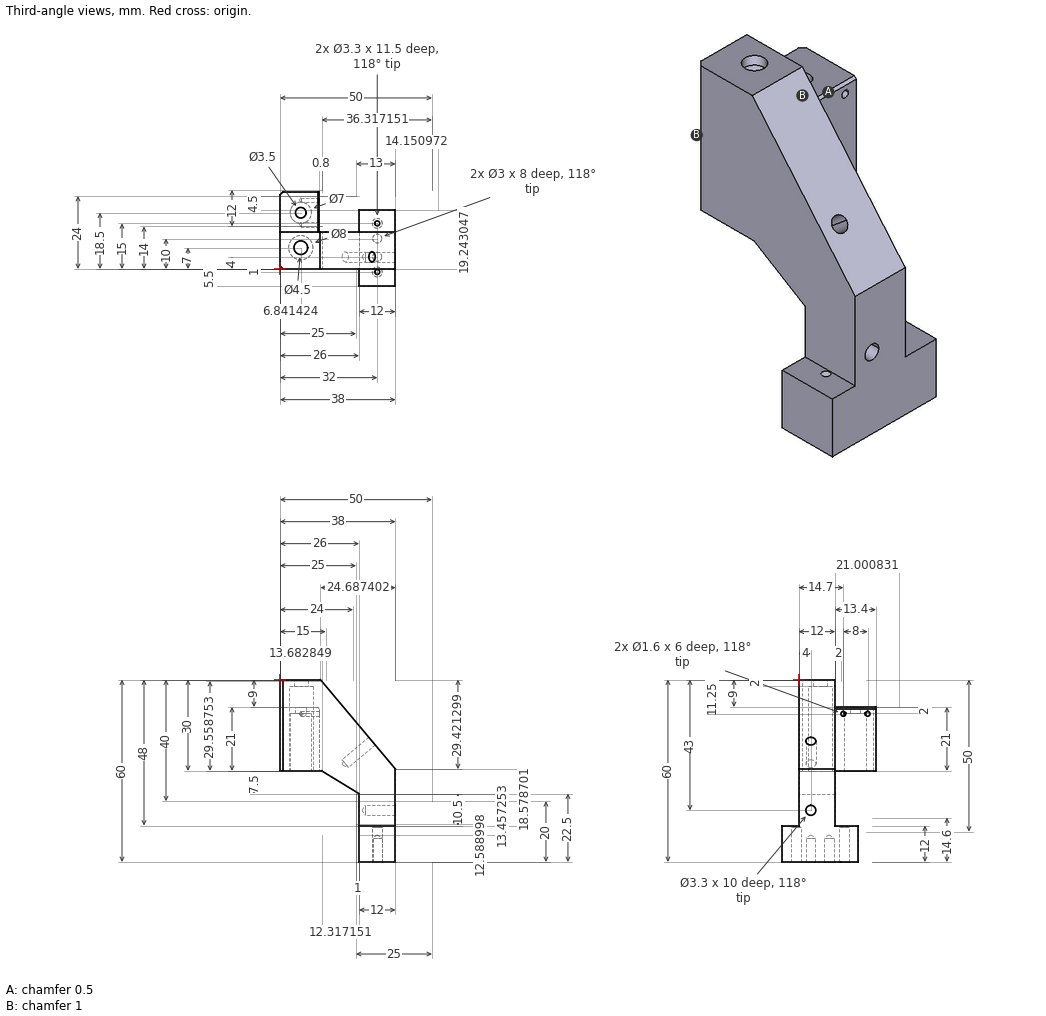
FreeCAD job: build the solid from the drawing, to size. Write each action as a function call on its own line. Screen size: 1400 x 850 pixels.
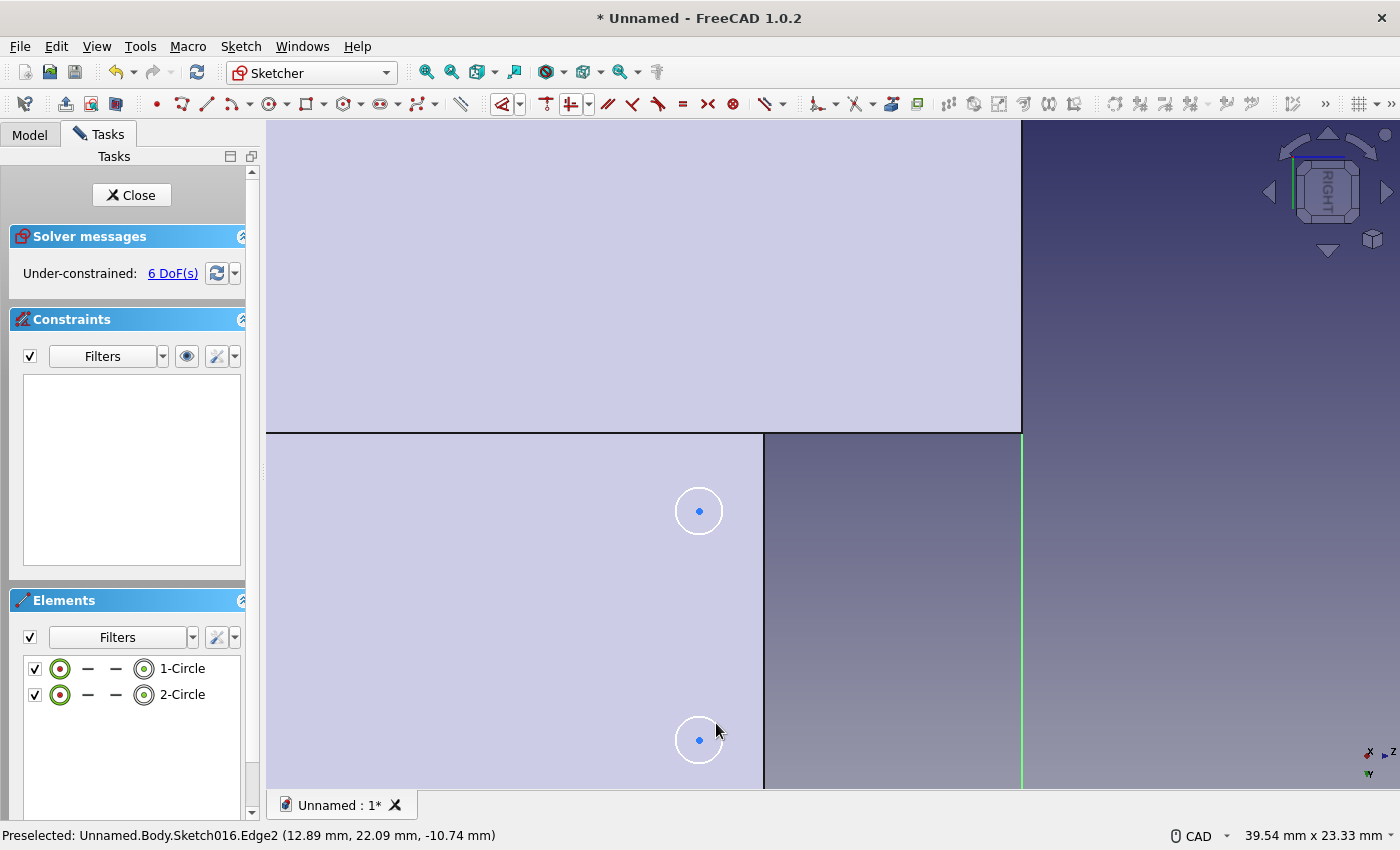
click(715, 494)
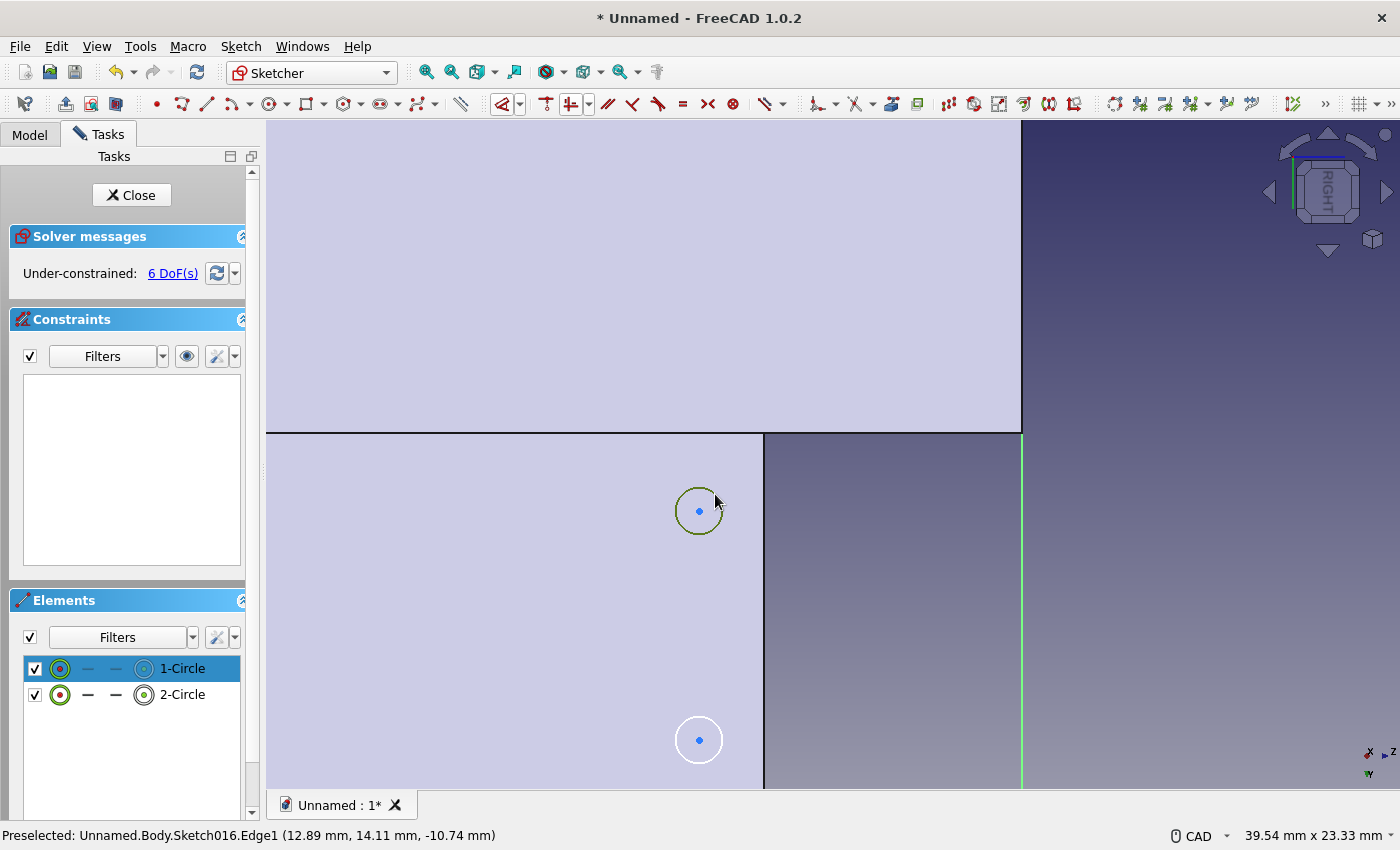
click(715, 723)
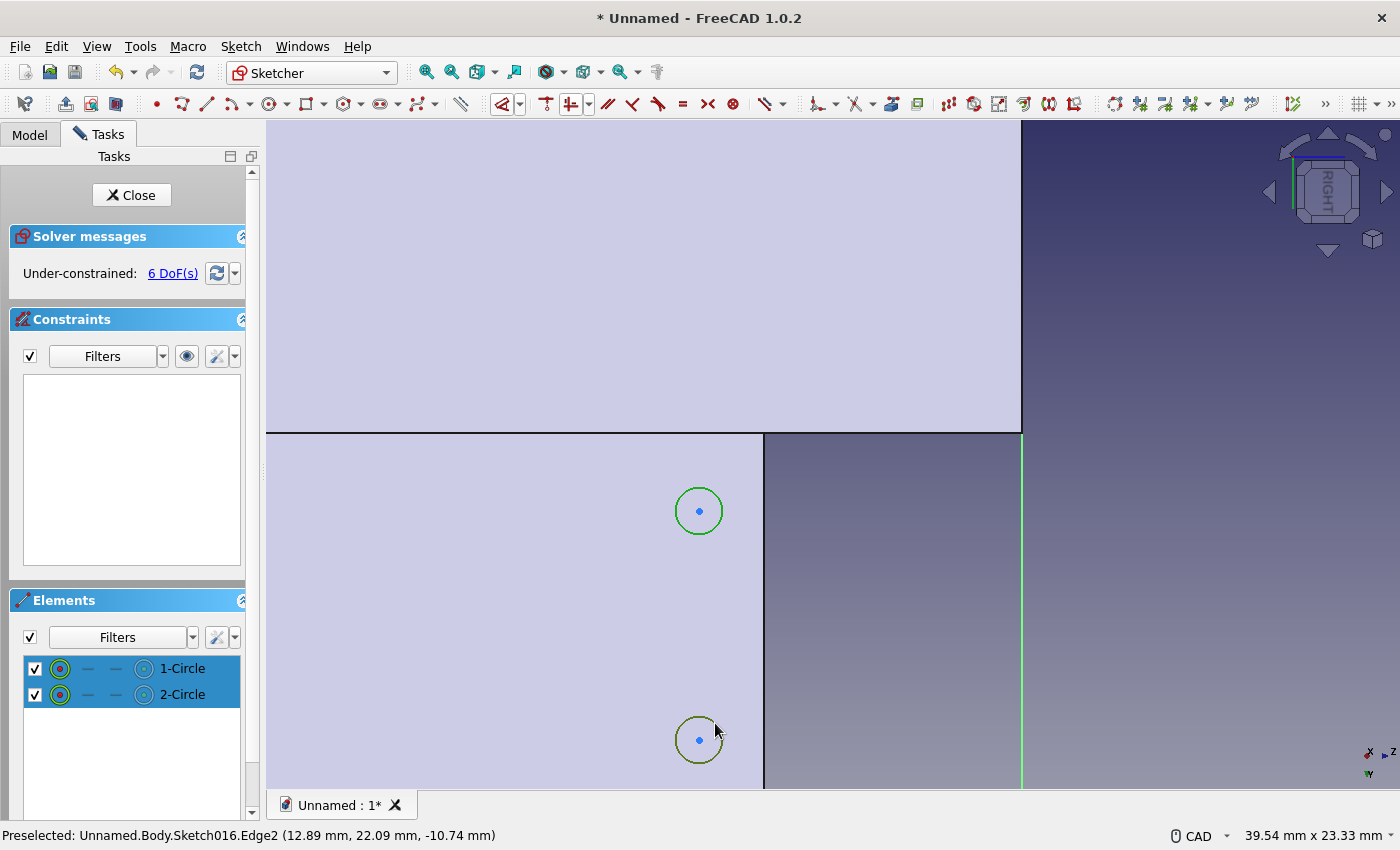
click(683, 104)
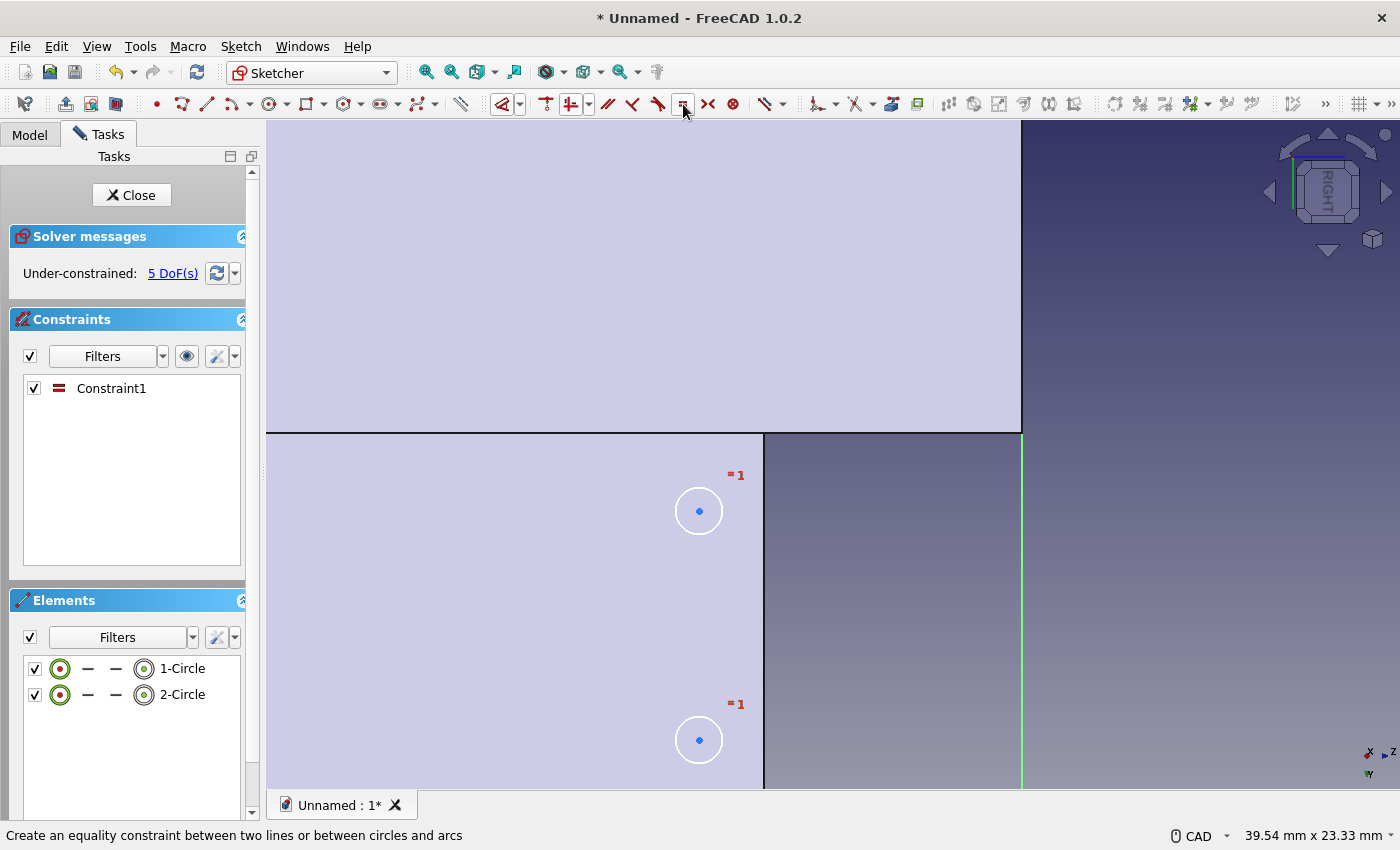
click(699, 511)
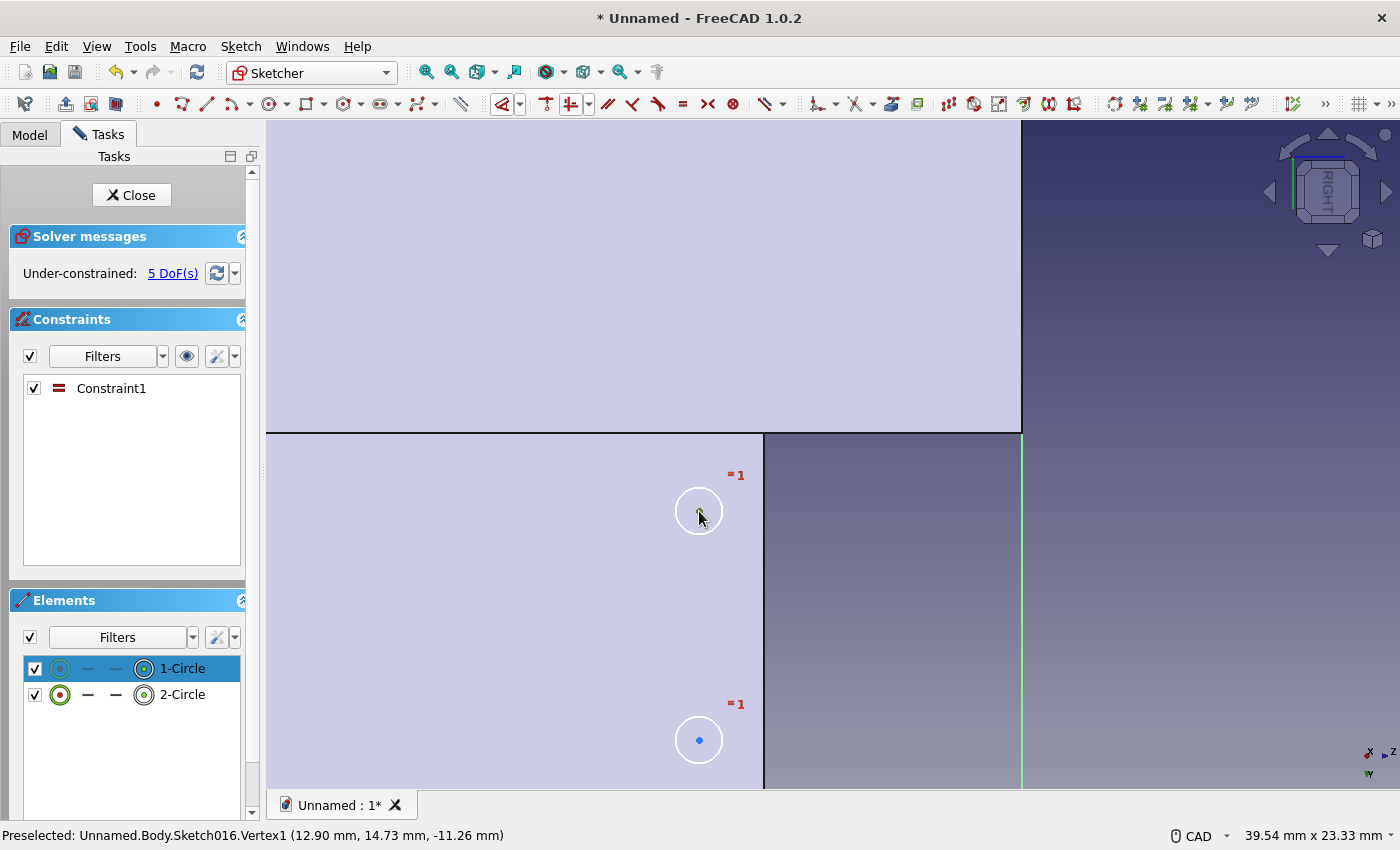
click(699, 740)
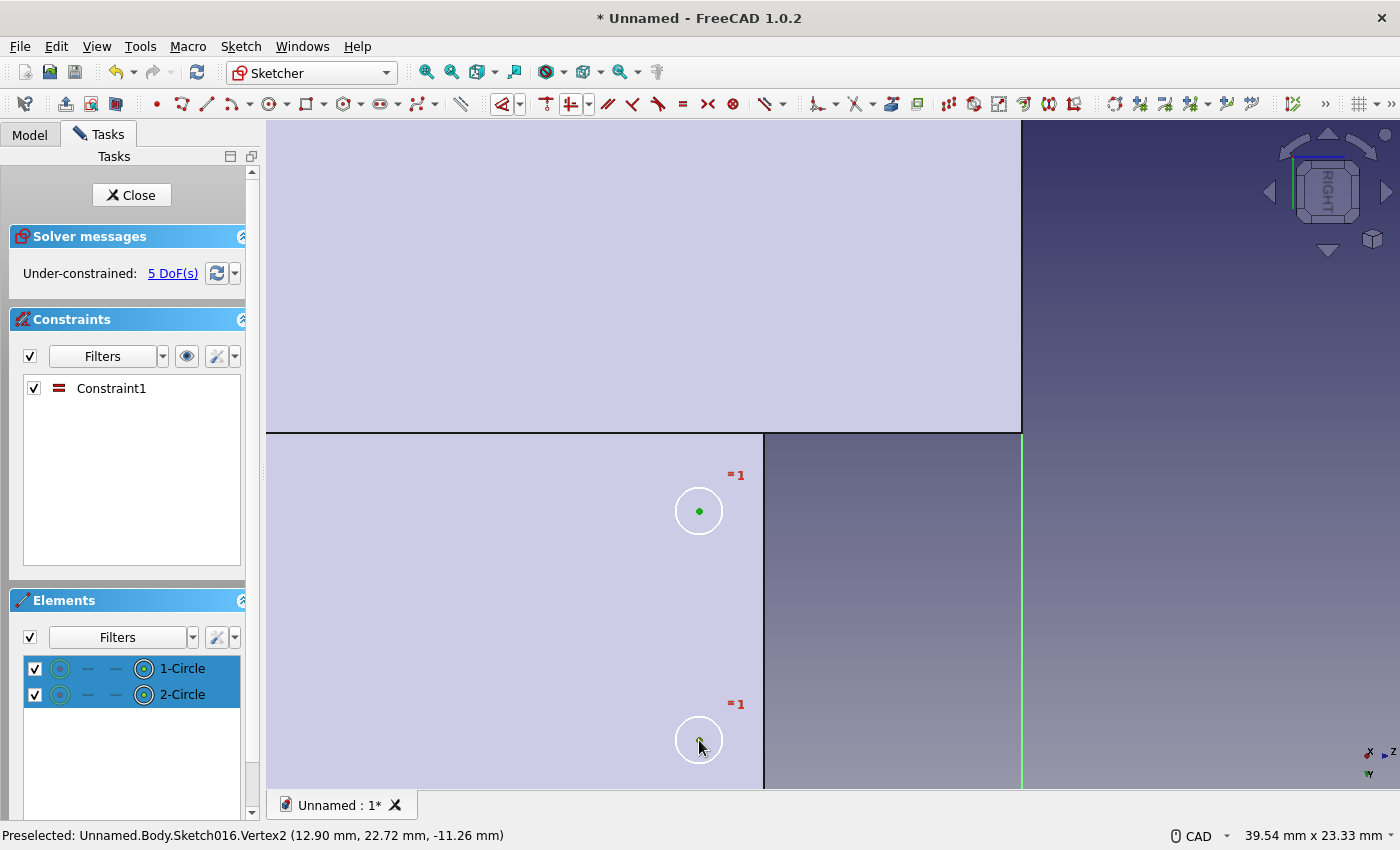
key(v)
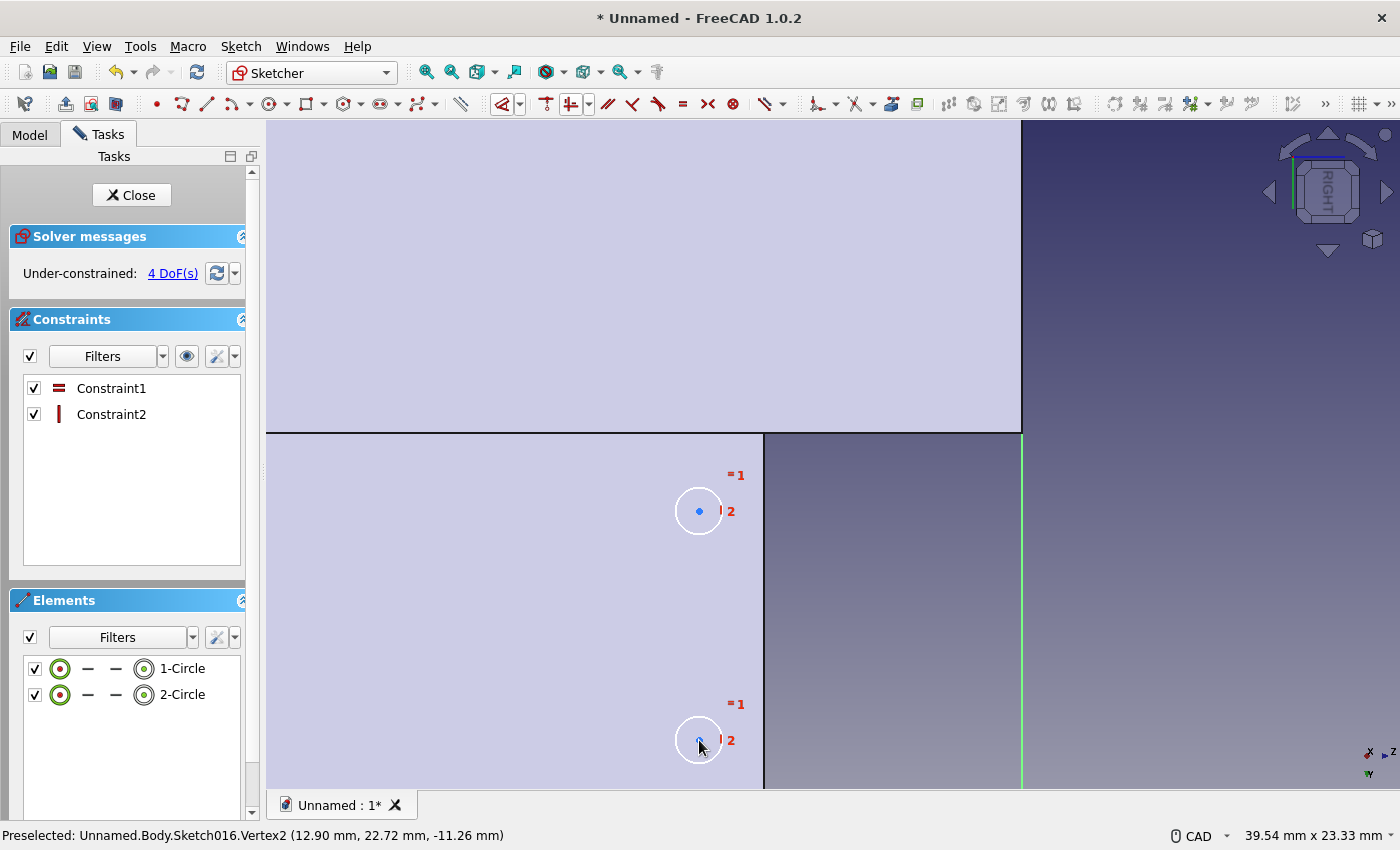
click(715, 494)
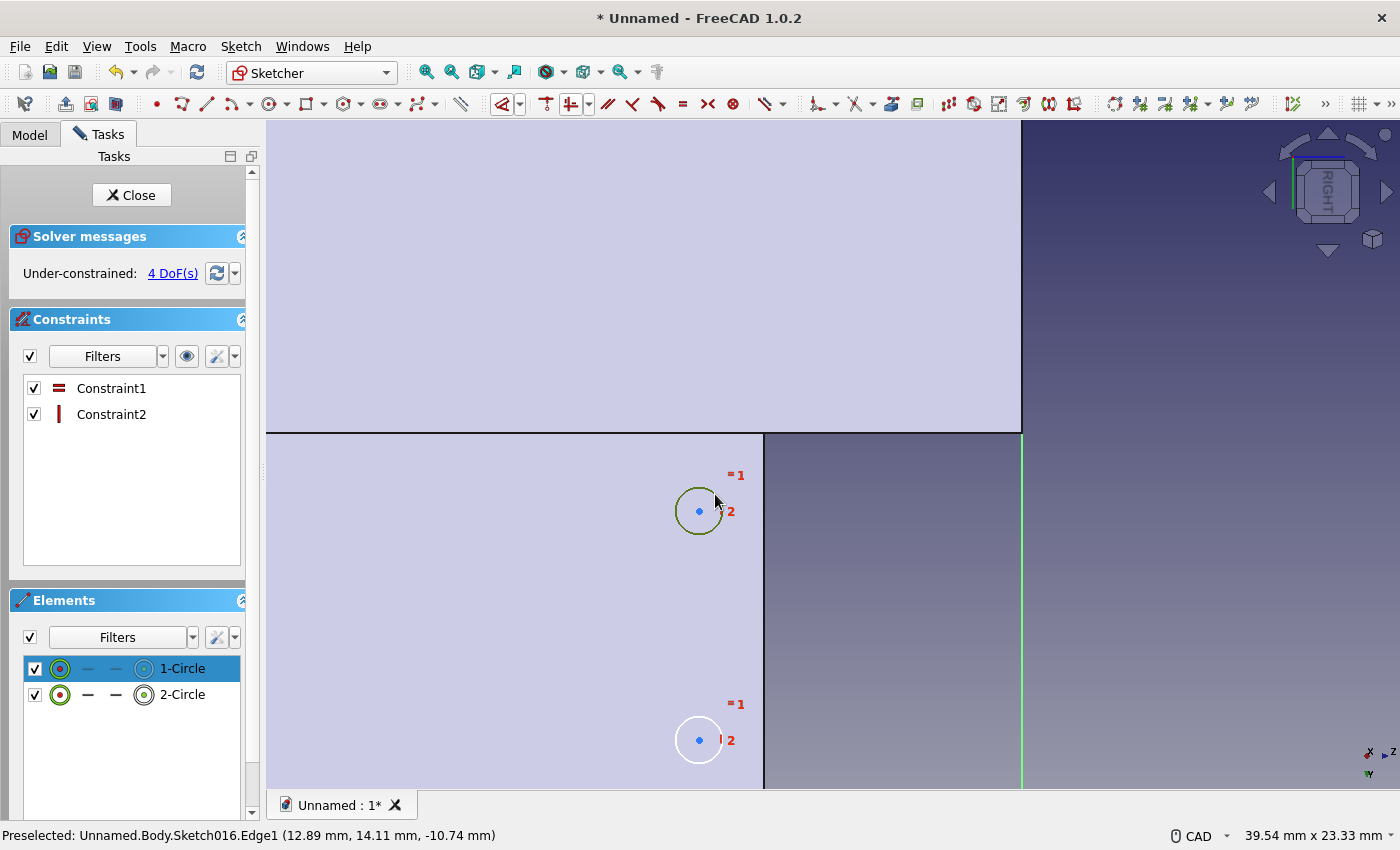
click(520, 104)